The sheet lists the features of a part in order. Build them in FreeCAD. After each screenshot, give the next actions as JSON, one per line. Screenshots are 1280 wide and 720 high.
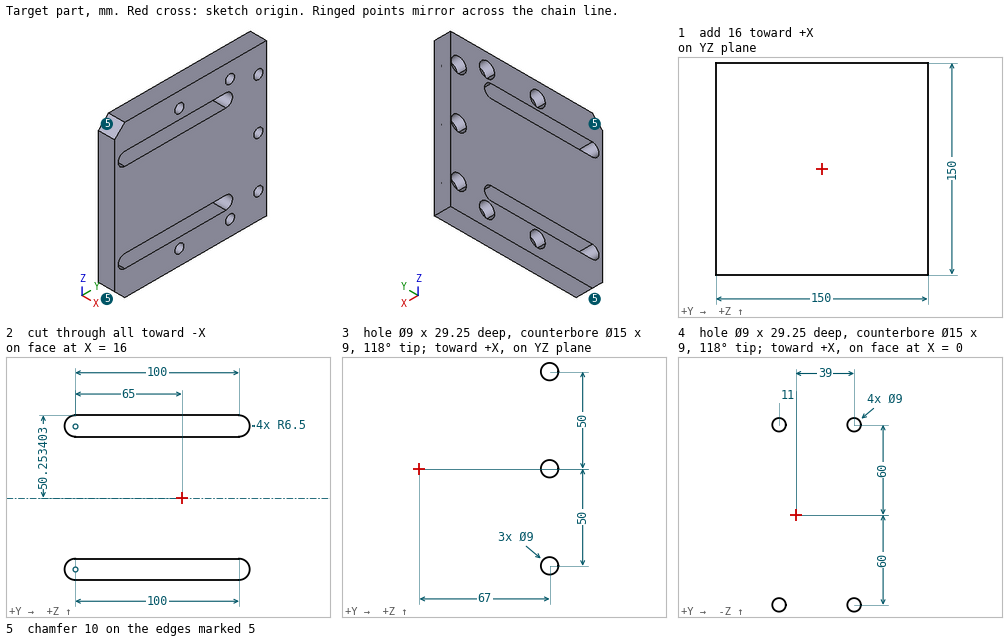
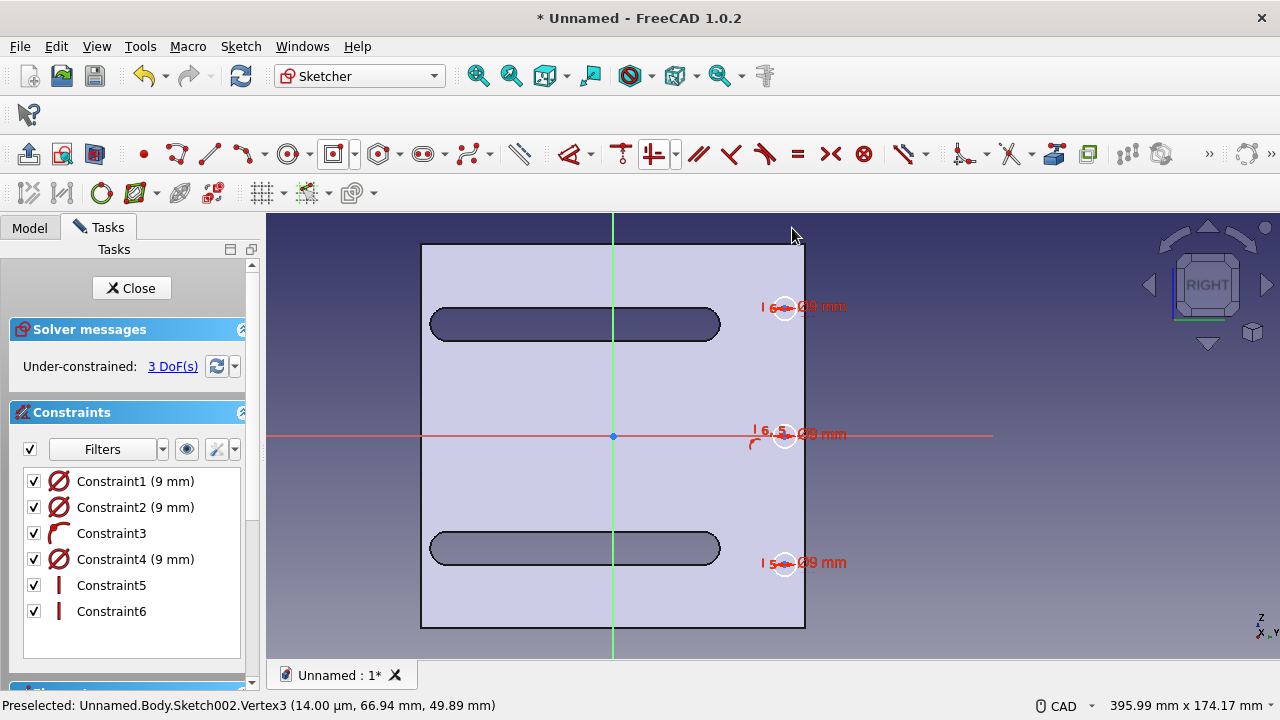
{"action": "left_click", "coordinate": [568, 154]}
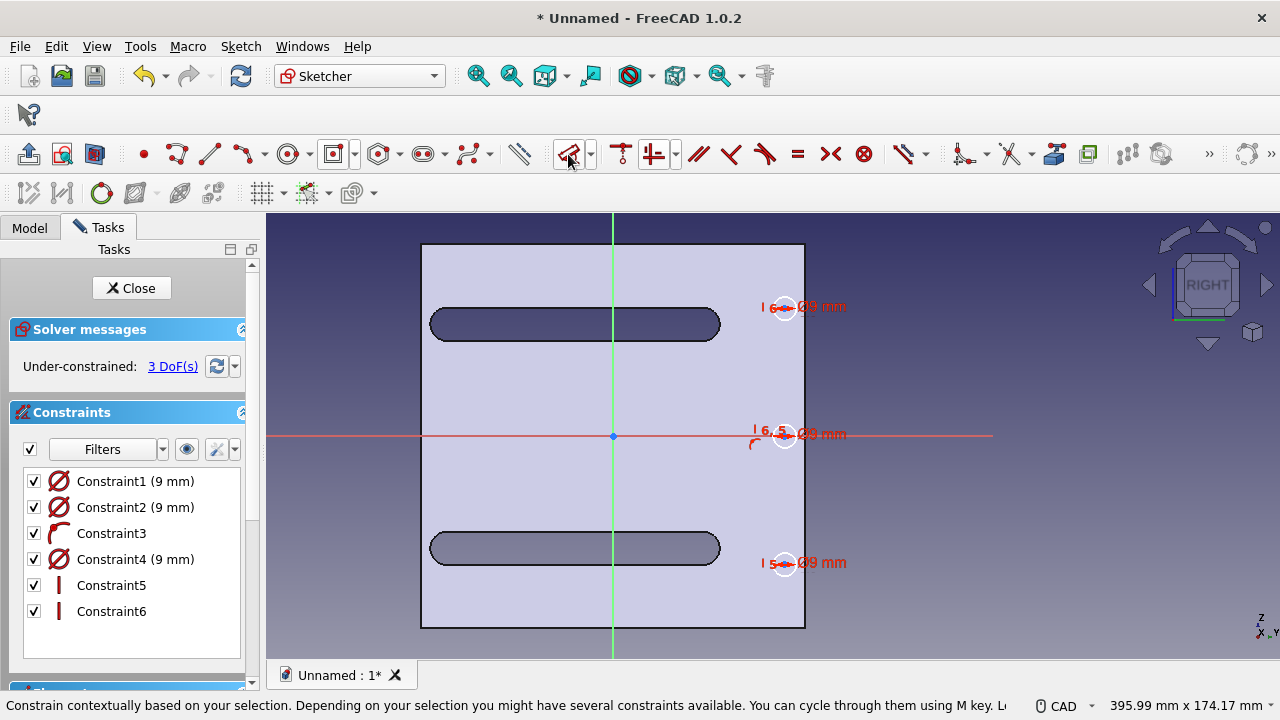
{"action": "left_click", "coordinate": [785, 565]}
{"action": "left_click", "coordinate": [699, 599]}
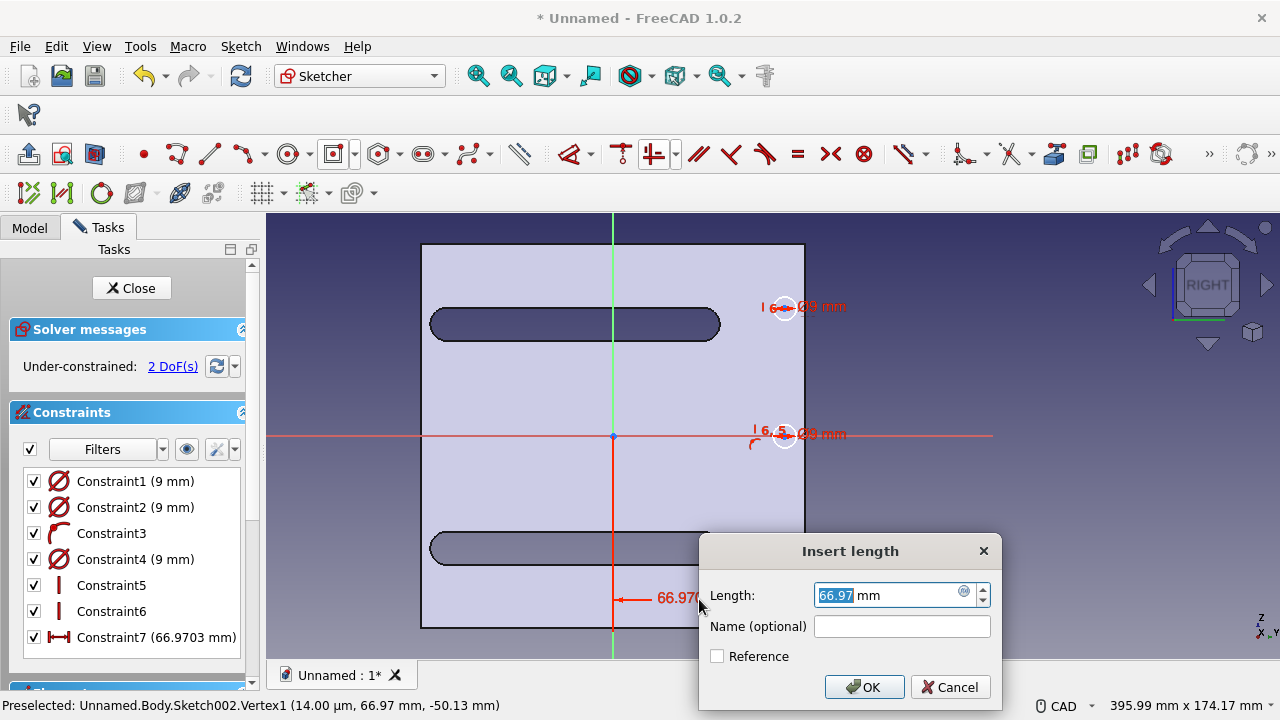
{"action": "type", "text": "67"}
{"action": "key", "text": "Return"}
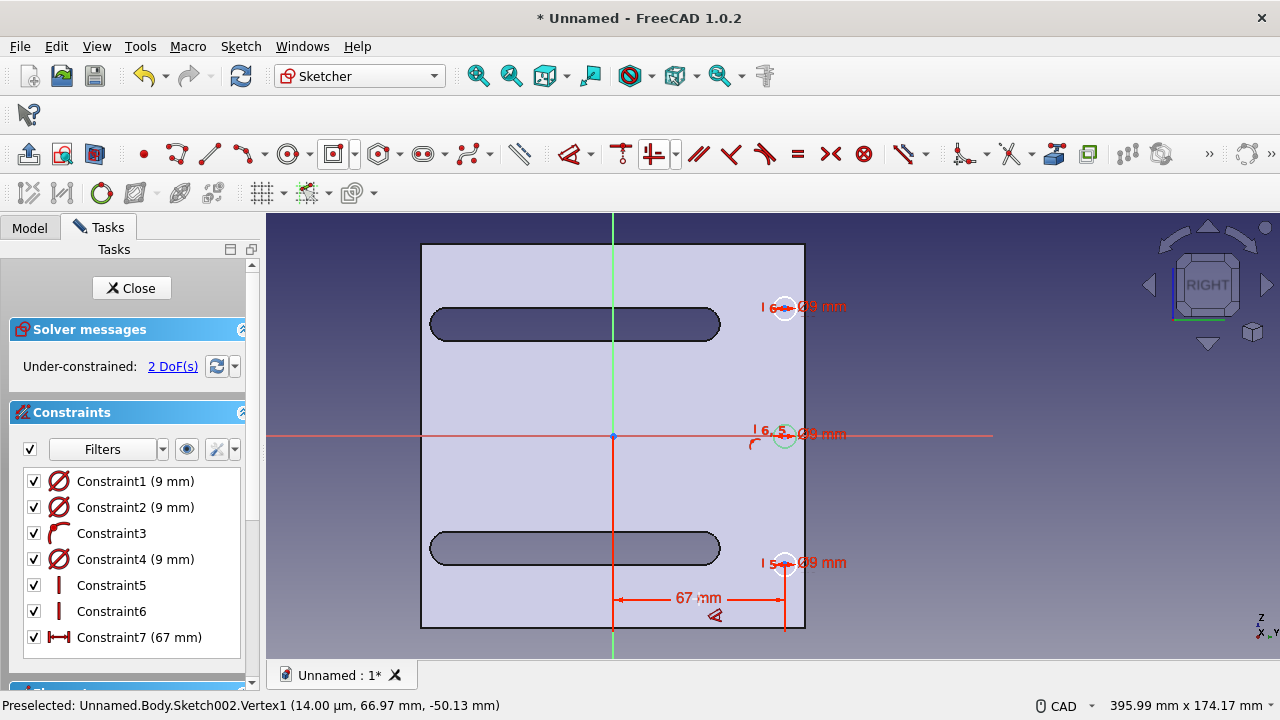
{"action": "left_click", "coordinate": [785, 565]}
{"action": "left_click", "coordinate": [579, 501]}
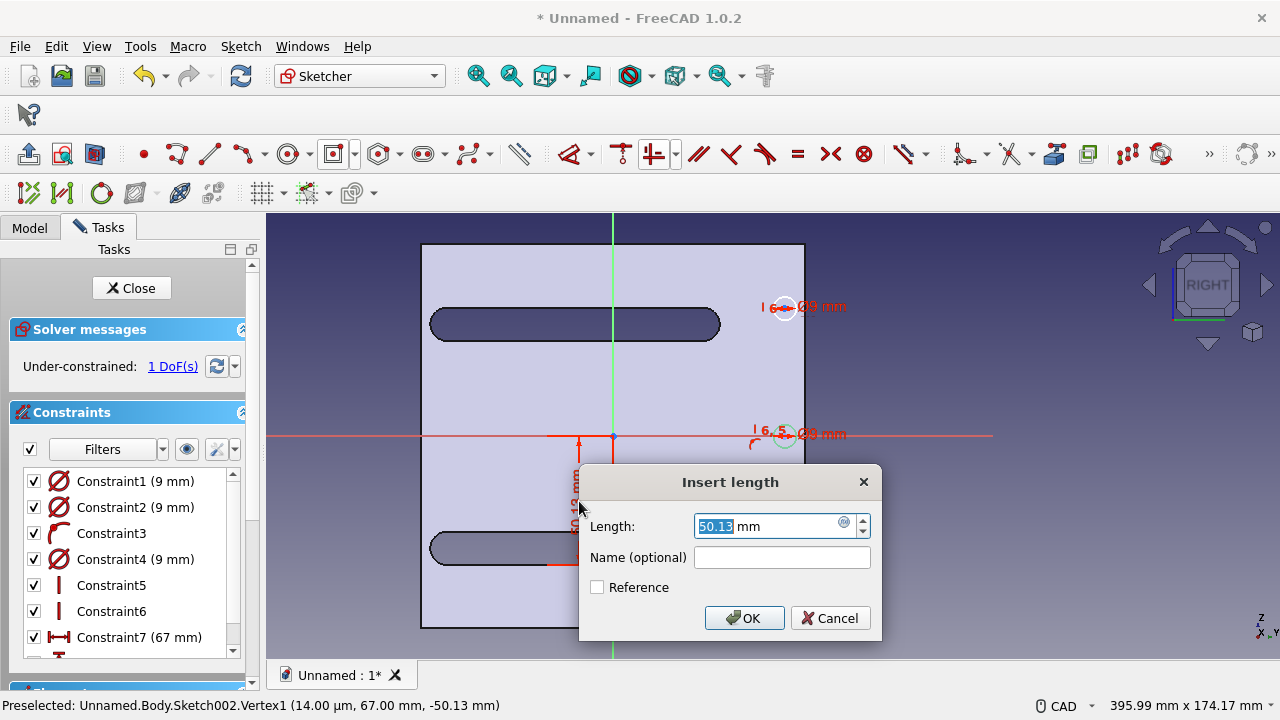
{"action": "type", "text": "50"}
{"action": "key", "text": "Return"}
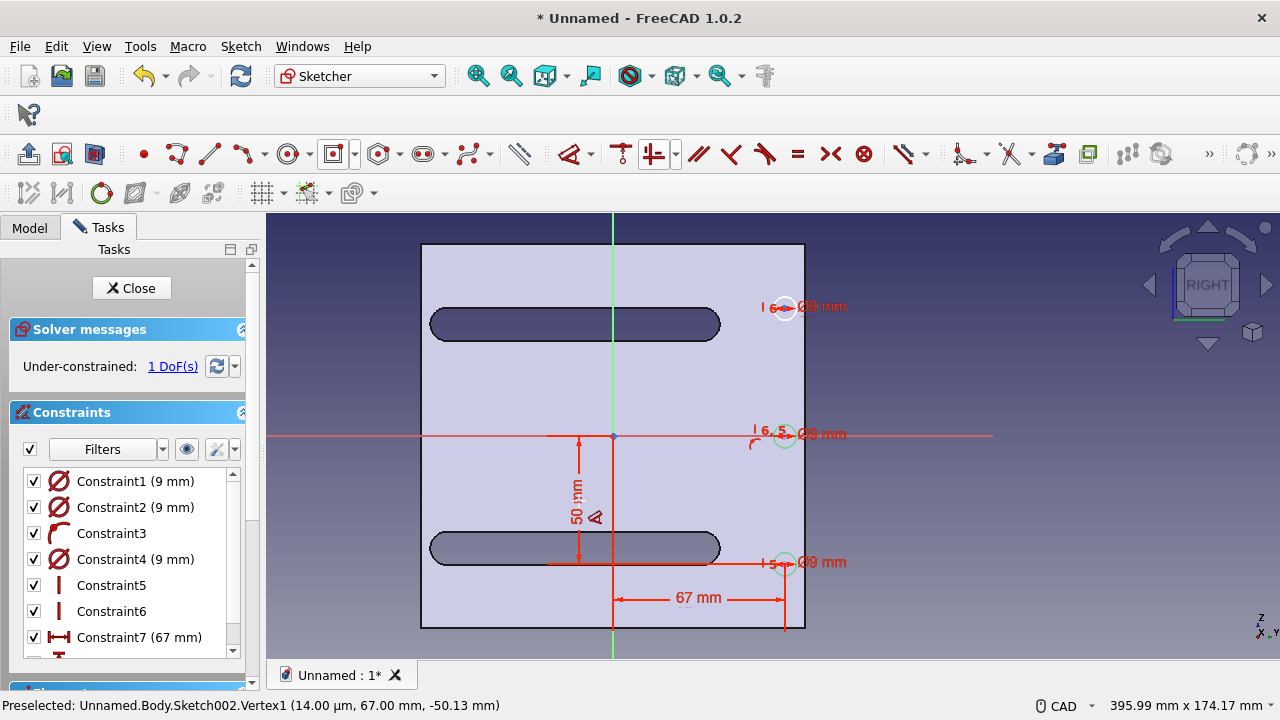
{"action": "left_click", "coordinate": [785, 309]}
{"action": "left_click", "coordinate": [579, 372]}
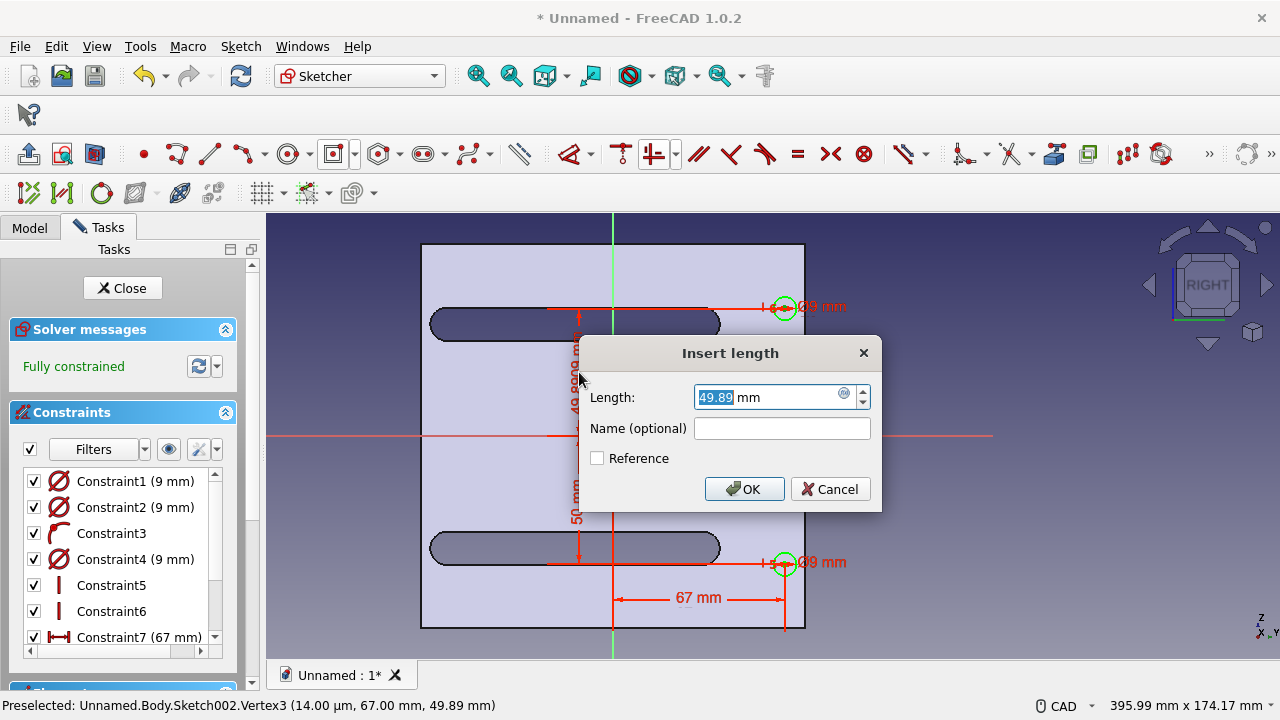
{"action": "type", "text": "50"}
{"action": "key", "text": "Return"}
{"action": "key", "text": "Escape"}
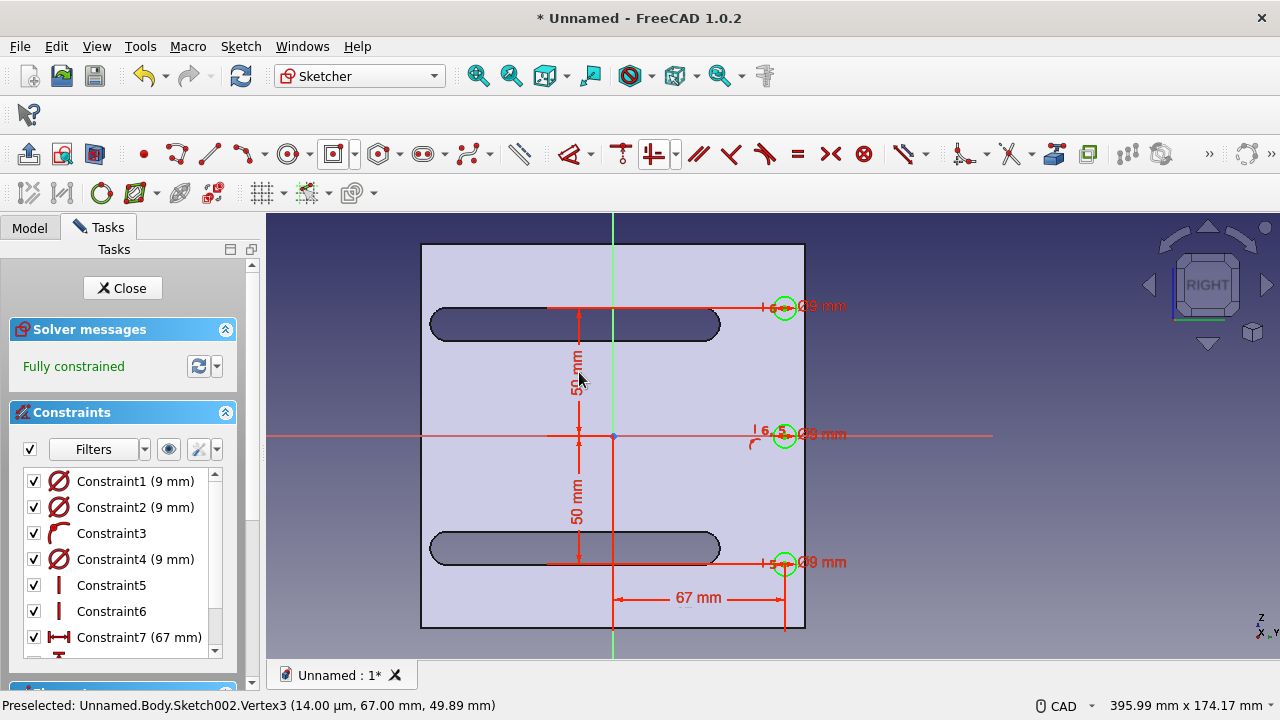
{"action": "left_click", "coordinate": [123, 288]}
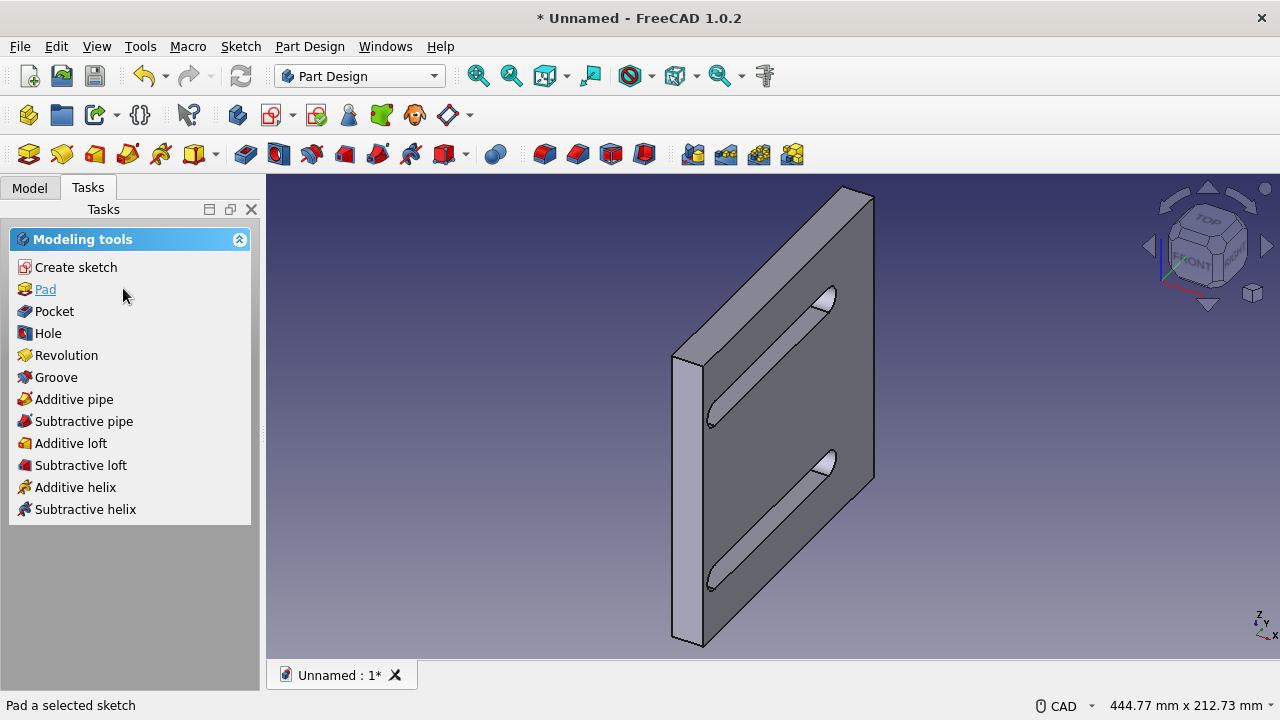
{"action": "left_click", "coordinate": [279, 154]}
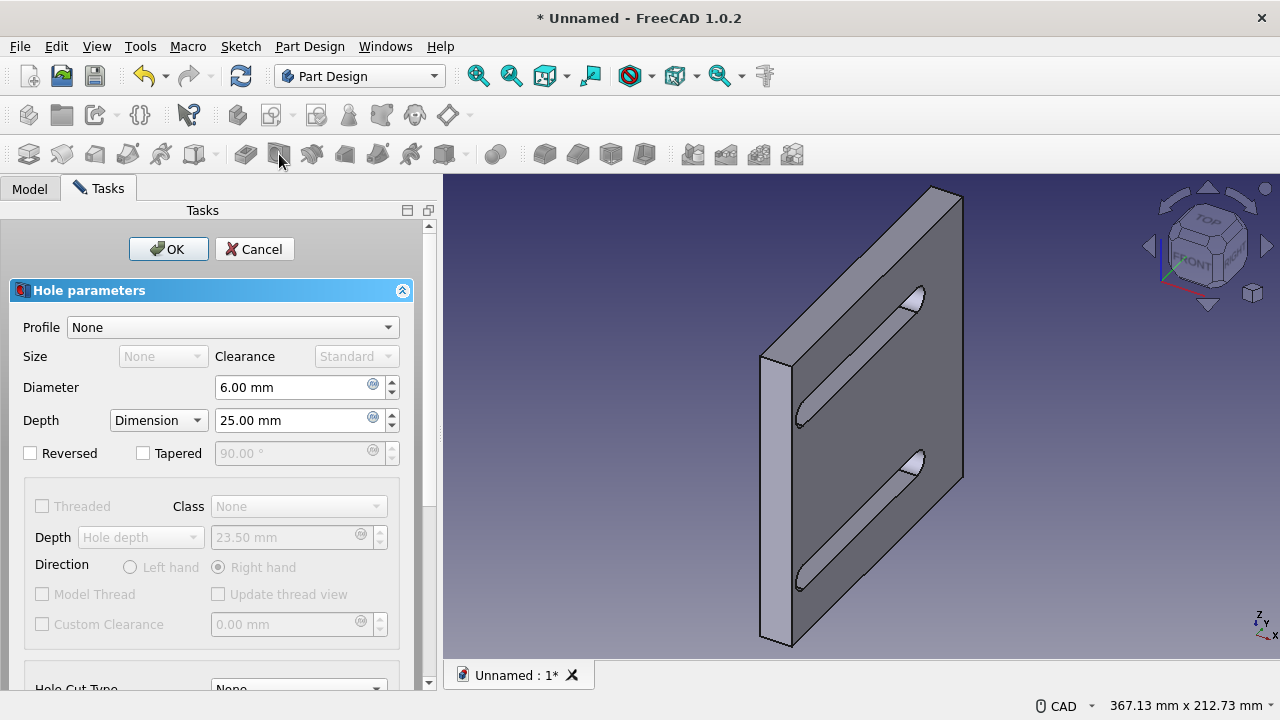
{"action": "triple_click", "coordinate": [300, 388]}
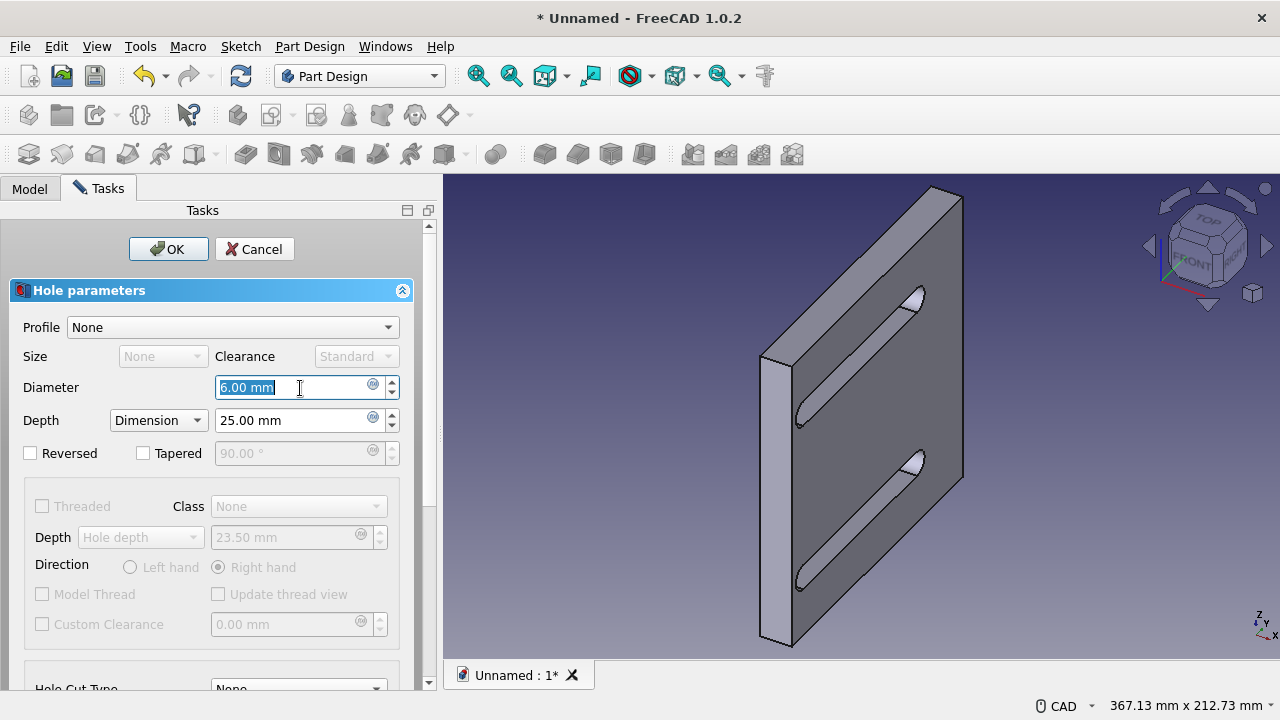
{"action": "type", "text": "9"}
{"action": "key", "text": "Tab"}